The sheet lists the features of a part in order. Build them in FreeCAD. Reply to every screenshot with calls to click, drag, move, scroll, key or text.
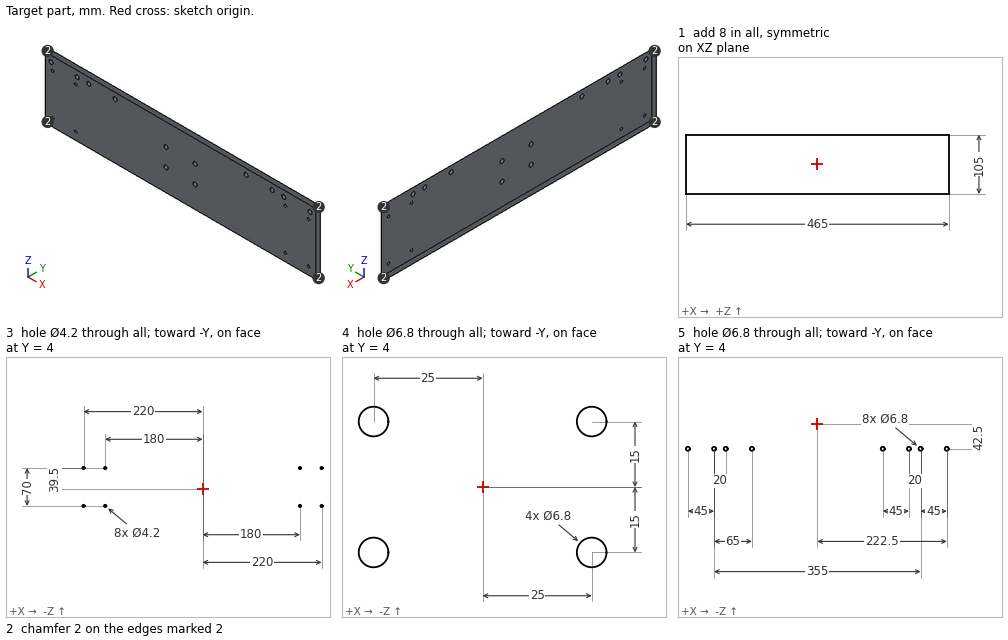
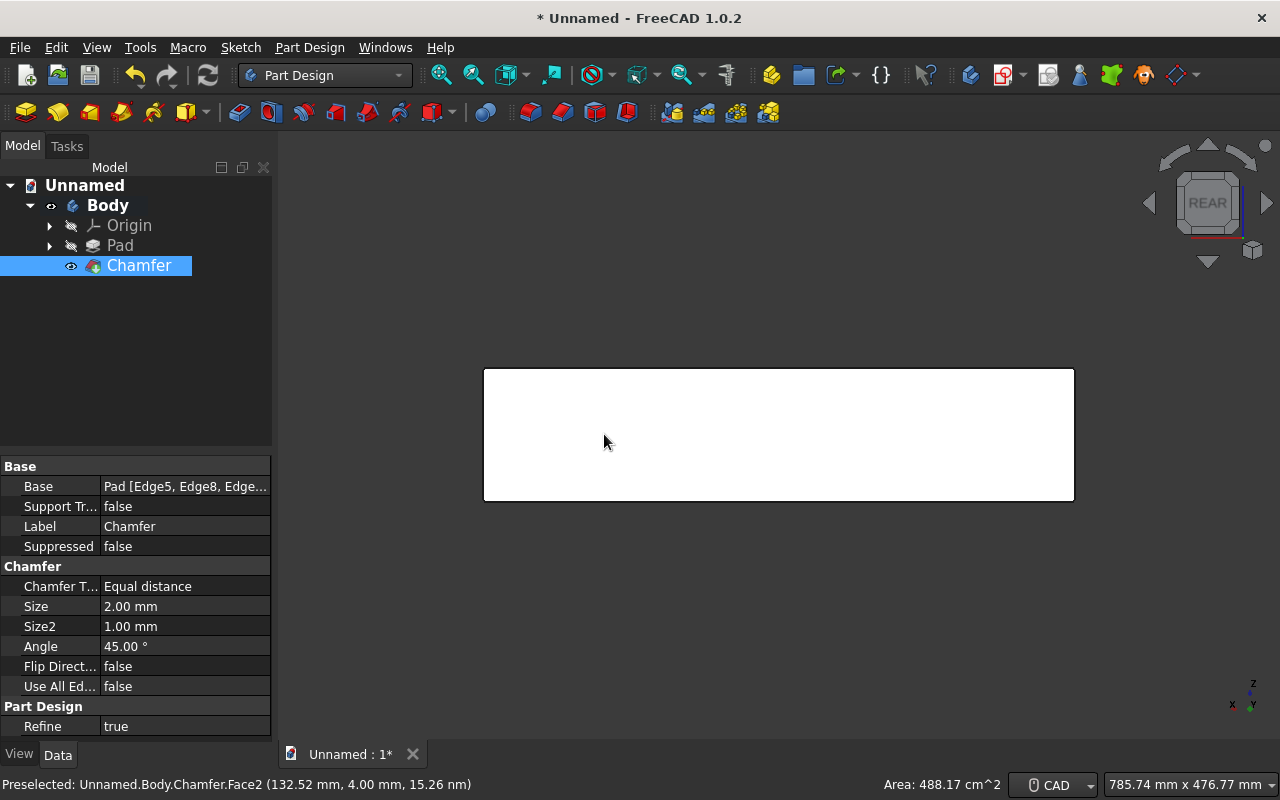
click(1004, 76)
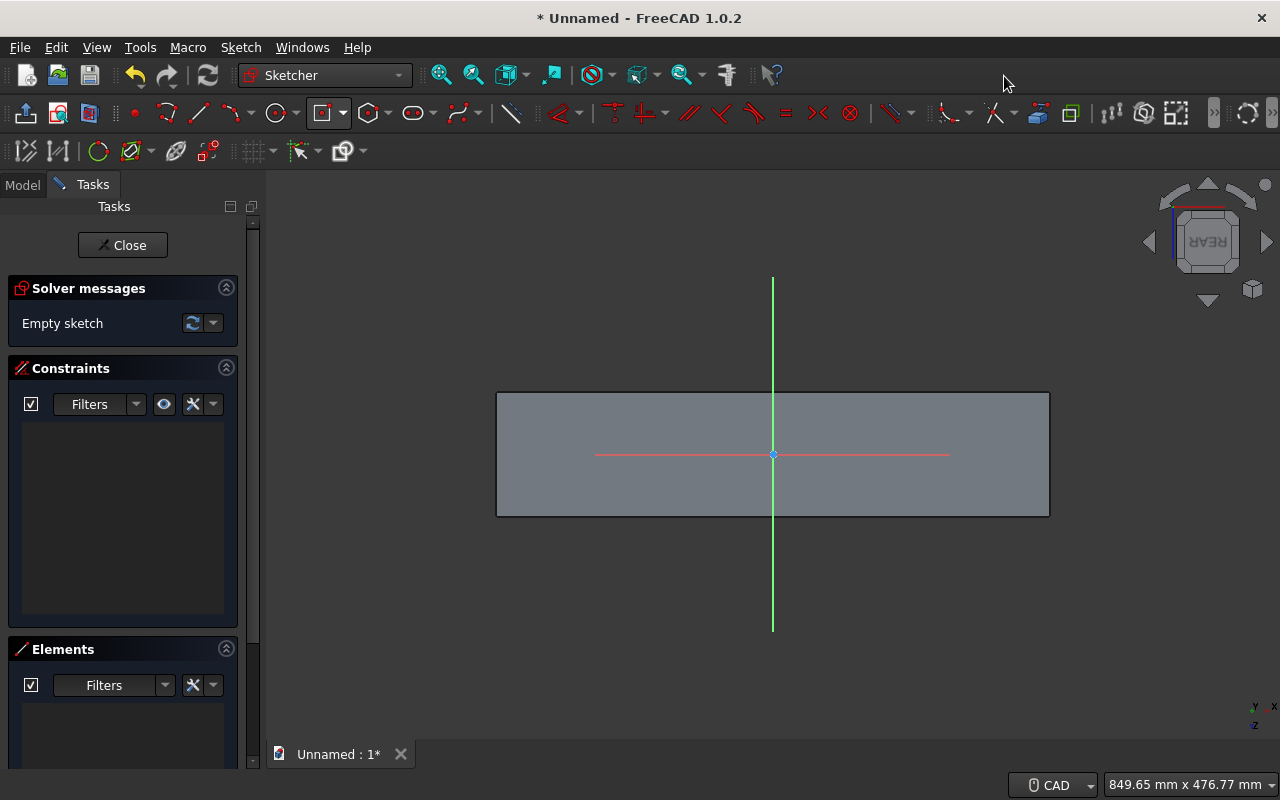
click(276, 114)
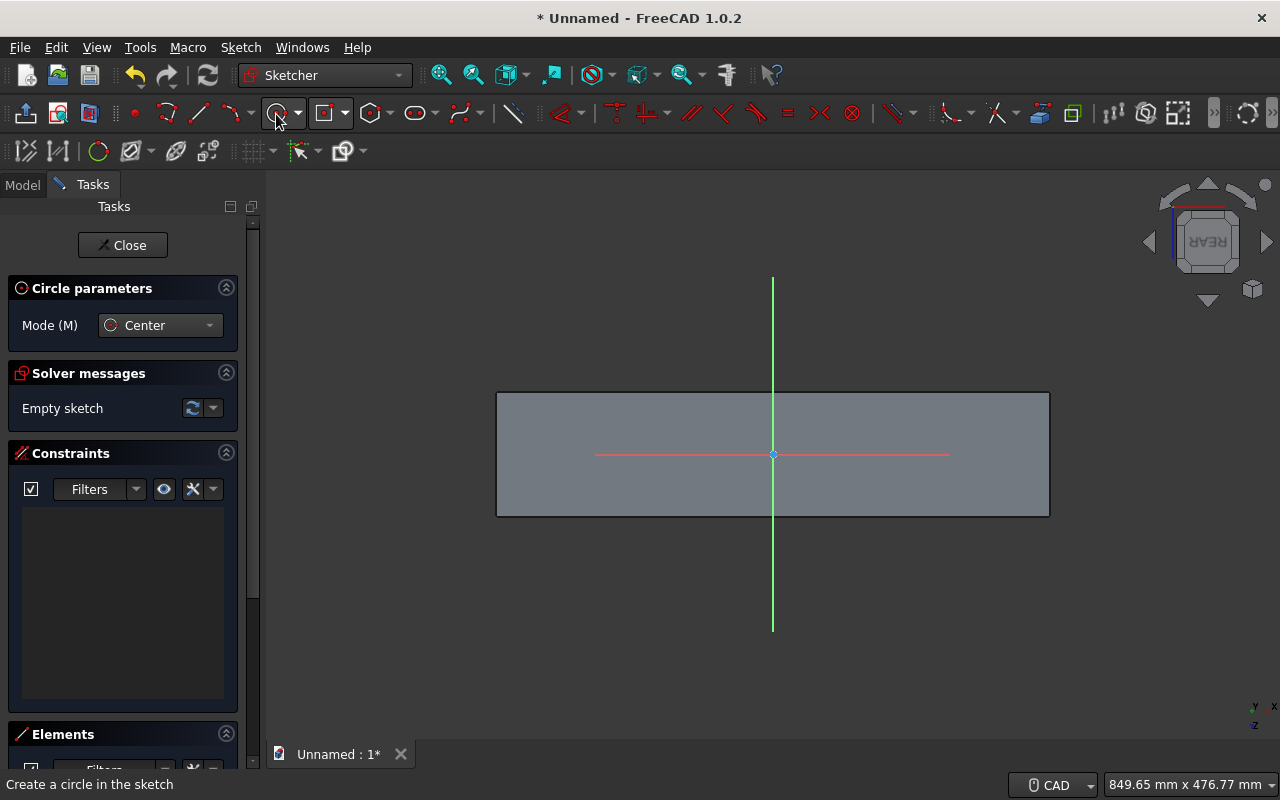
scroll(510, 407, up, 12)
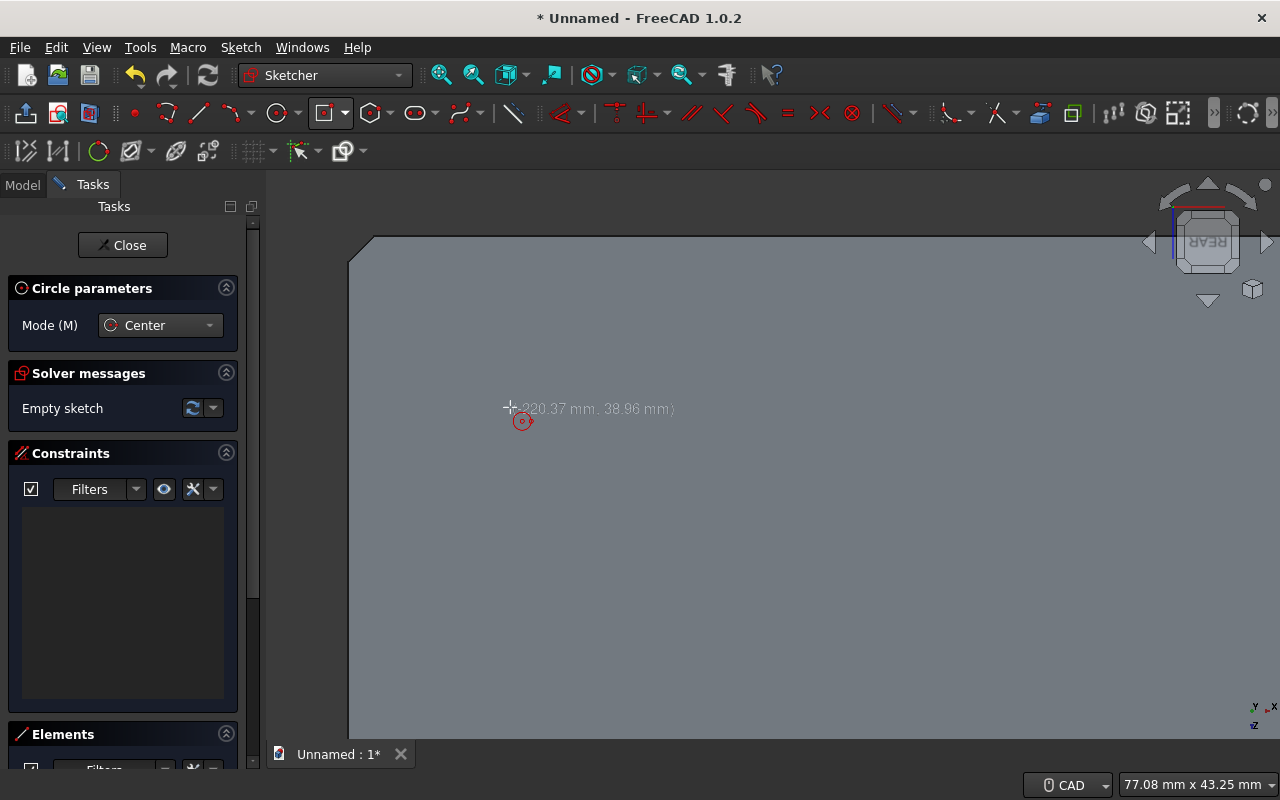
scroll(435, 413, down, 12)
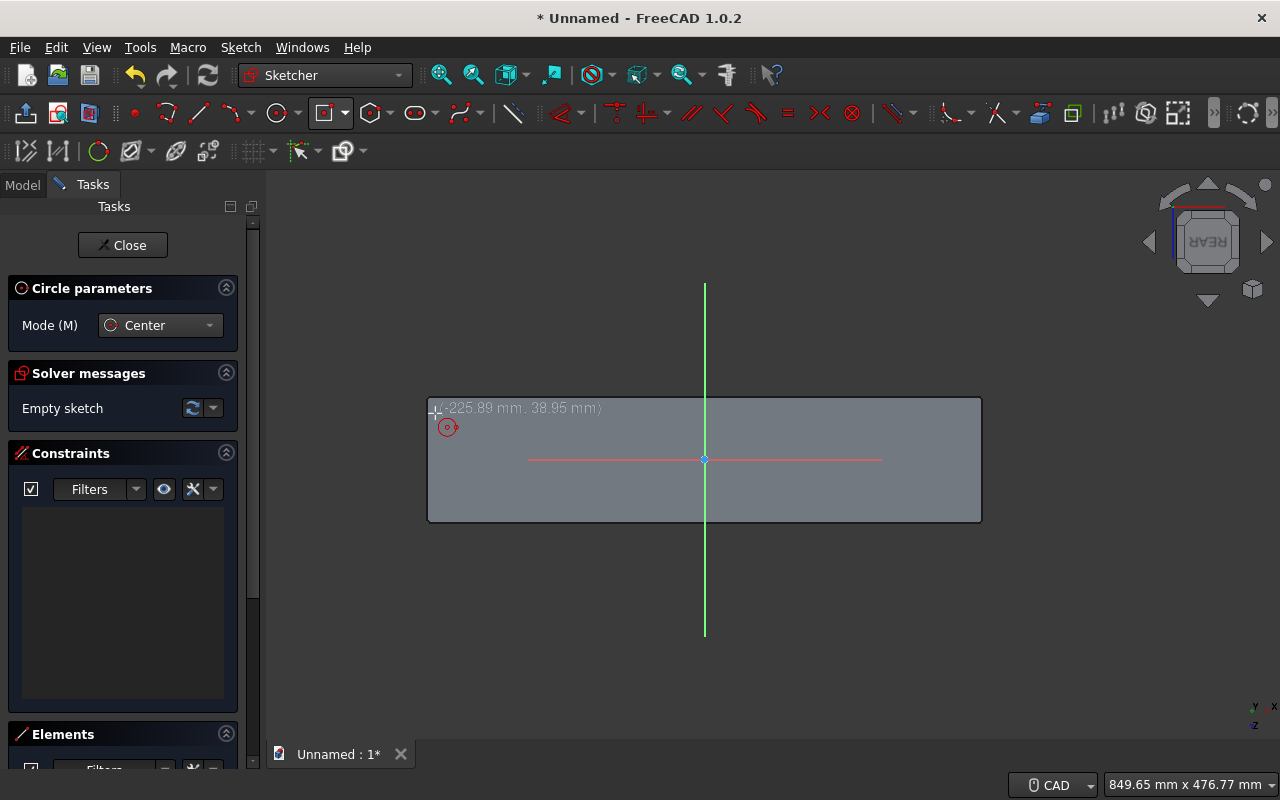
click(442, 413)
move(444, 411)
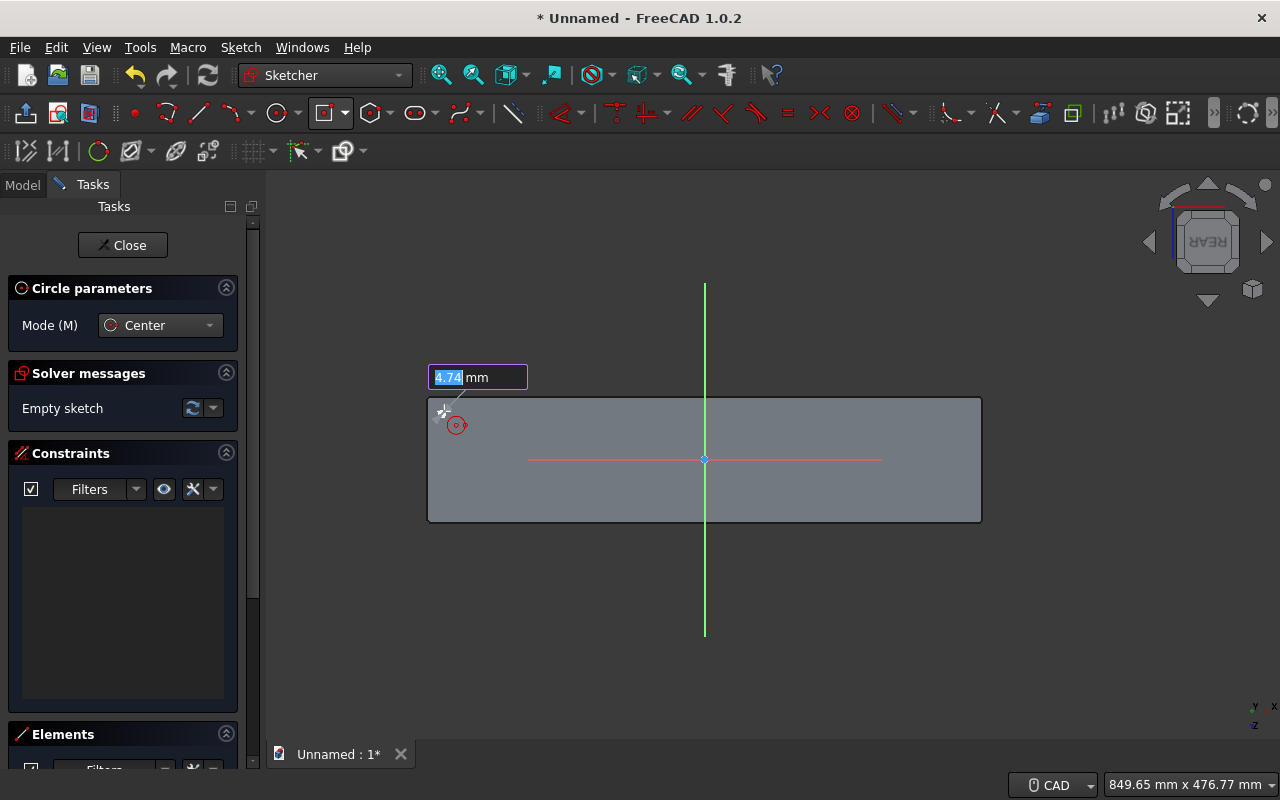
text(4.2)
key(Return)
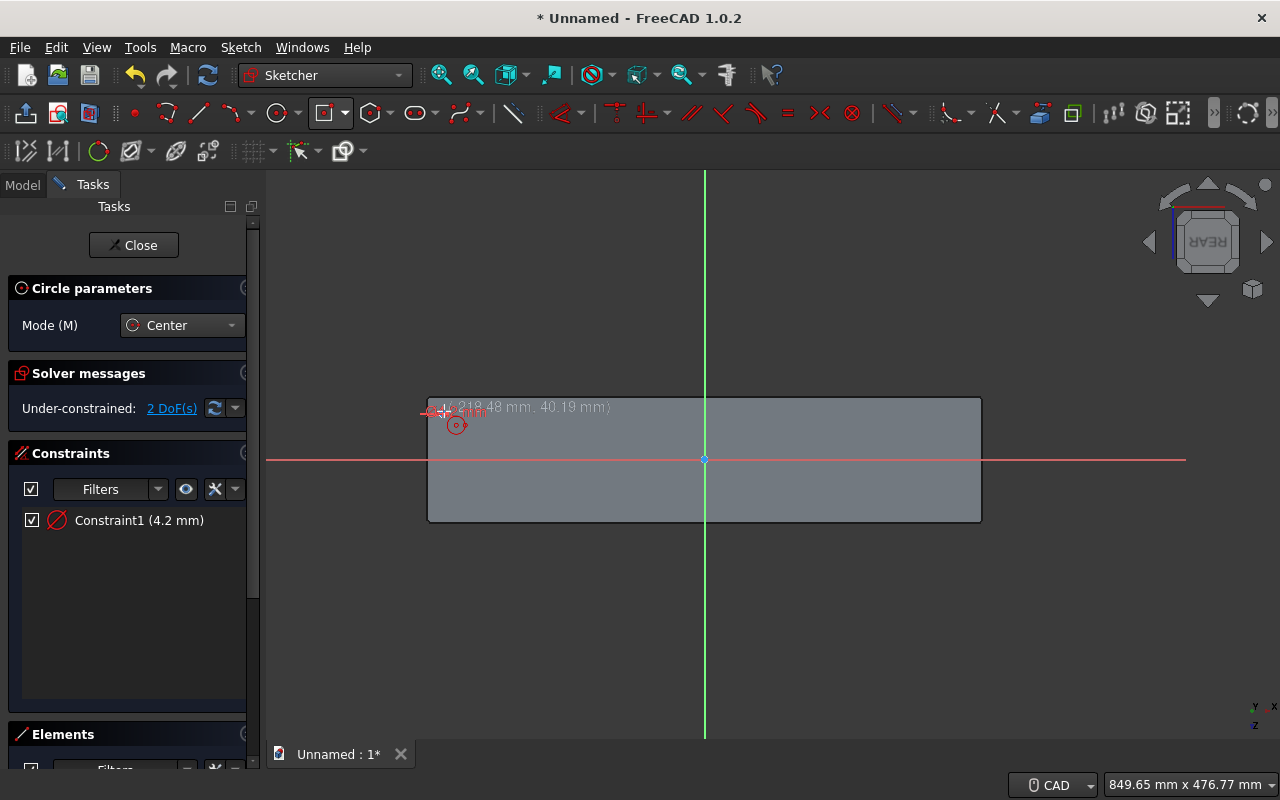
scroll(490, 413, up, 12)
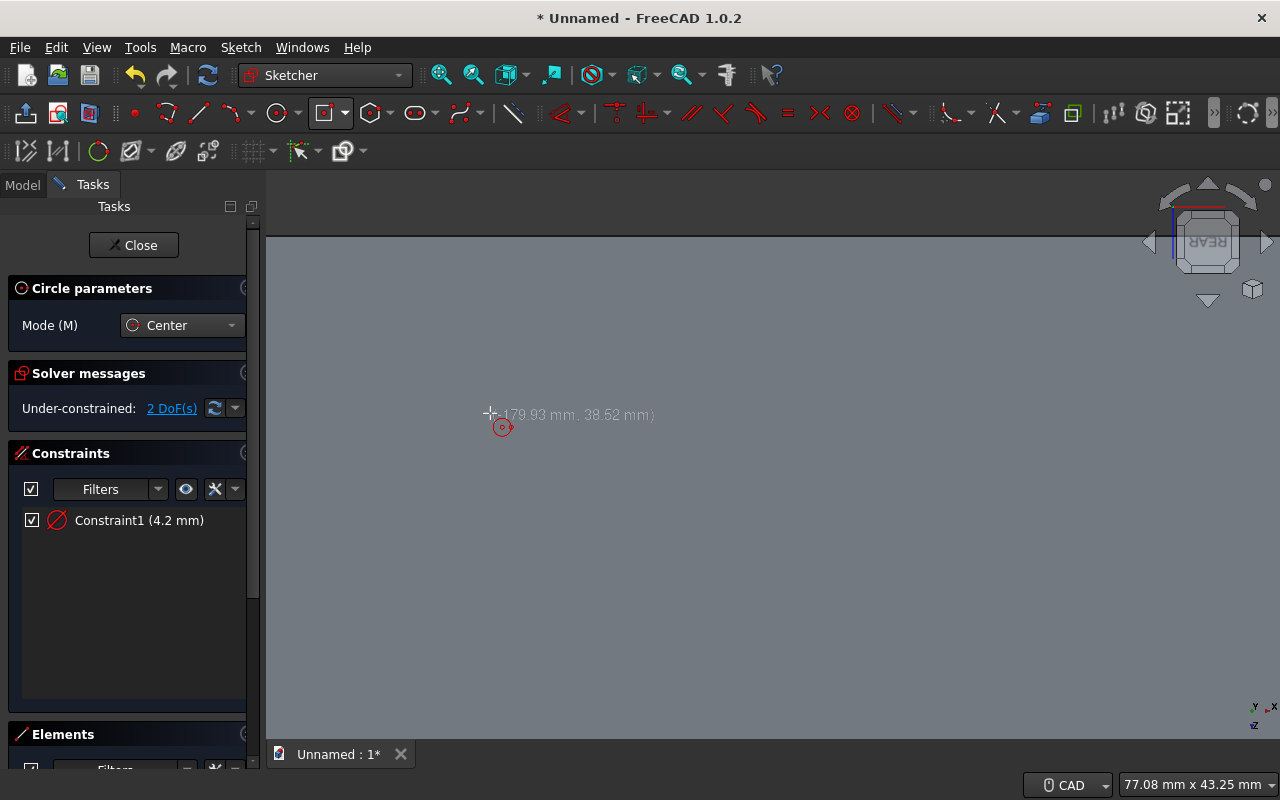
scroll(490, 413, down, 12)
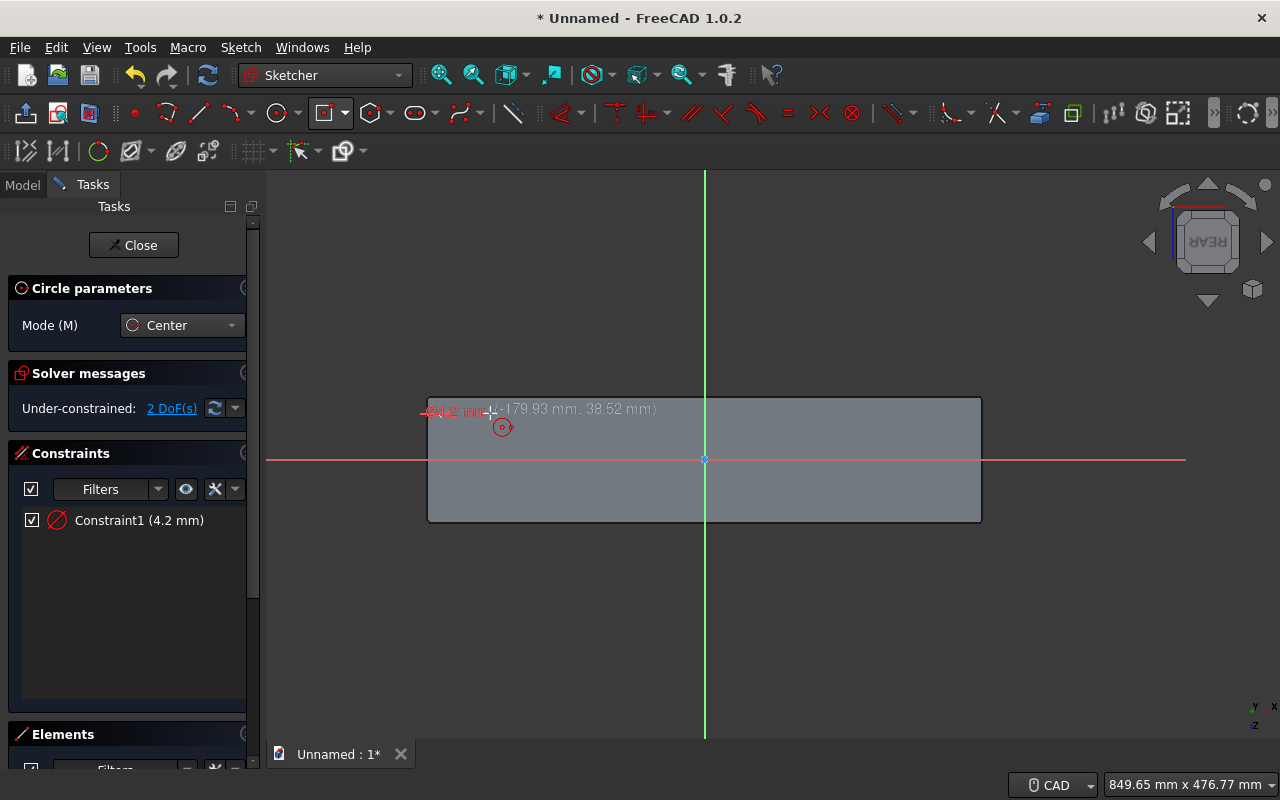
click(490, 413)
move(492, 411)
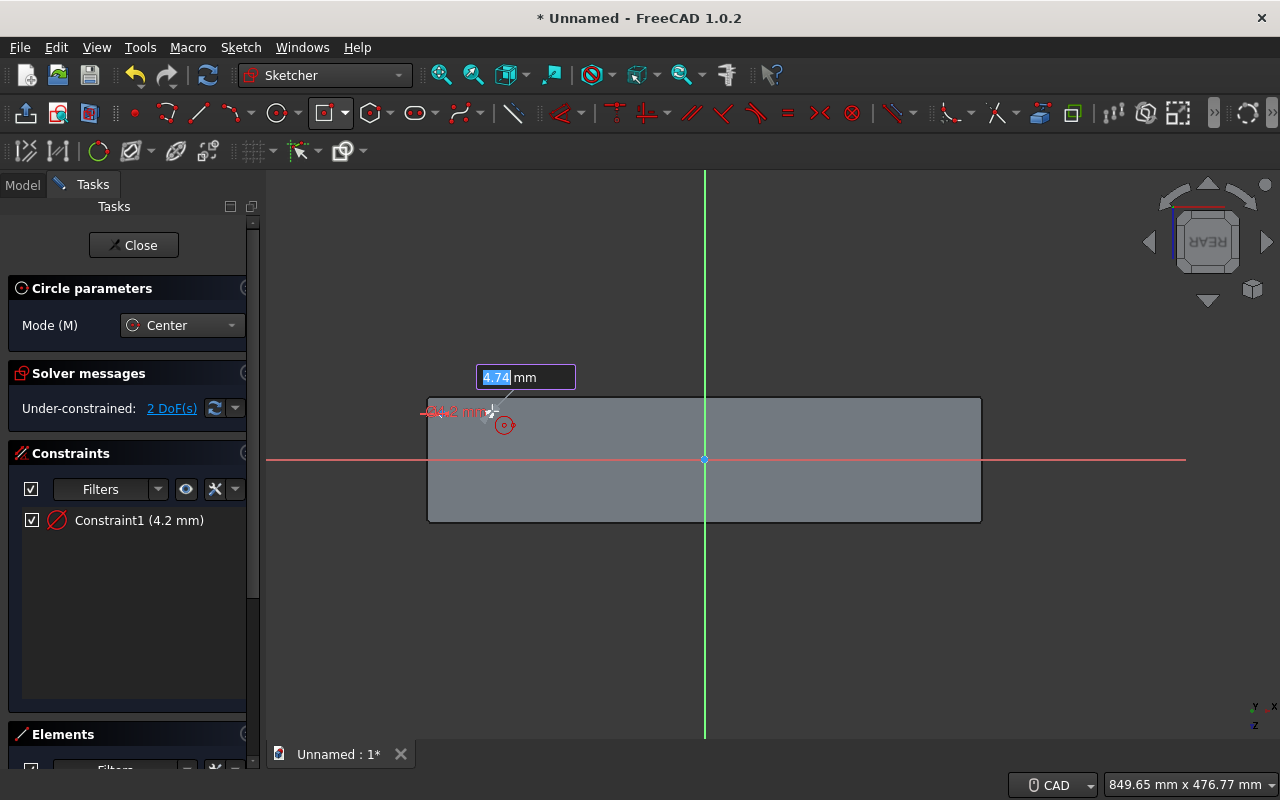
text(4.2)
key(Return)